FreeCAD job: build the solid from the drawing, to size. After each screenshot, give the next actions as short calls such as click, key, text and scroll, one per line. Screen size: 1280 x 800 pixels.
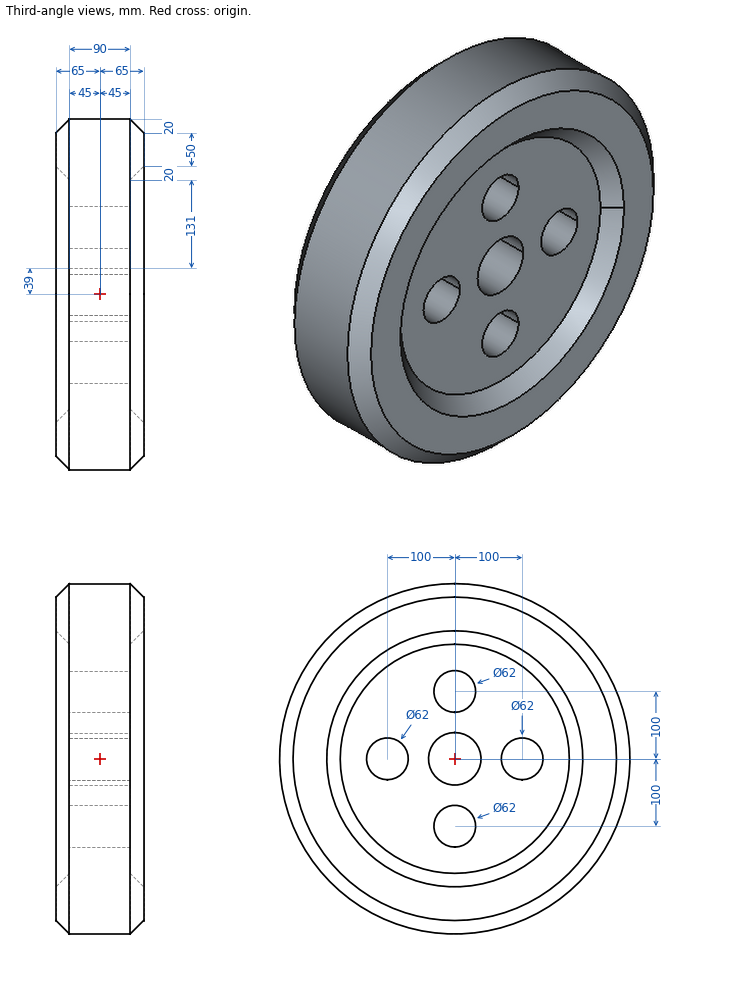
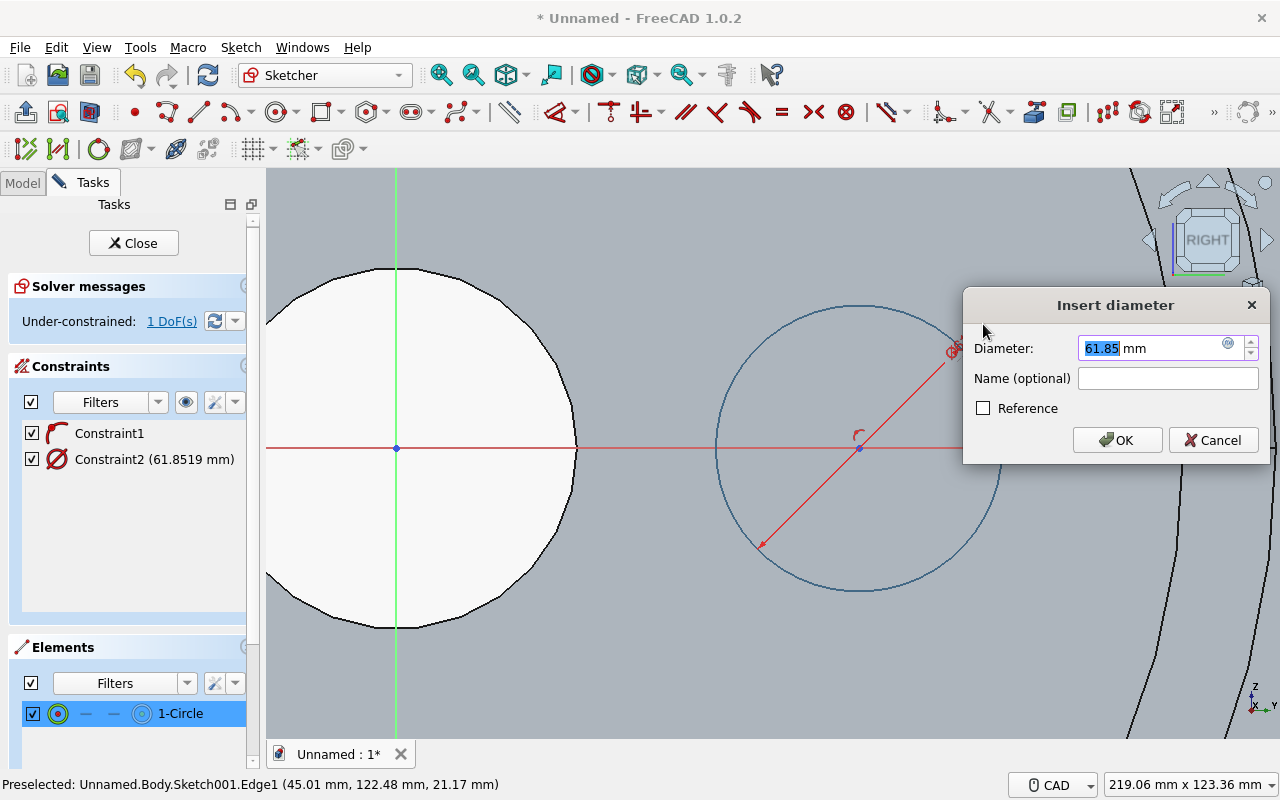
text(62)
key(Return)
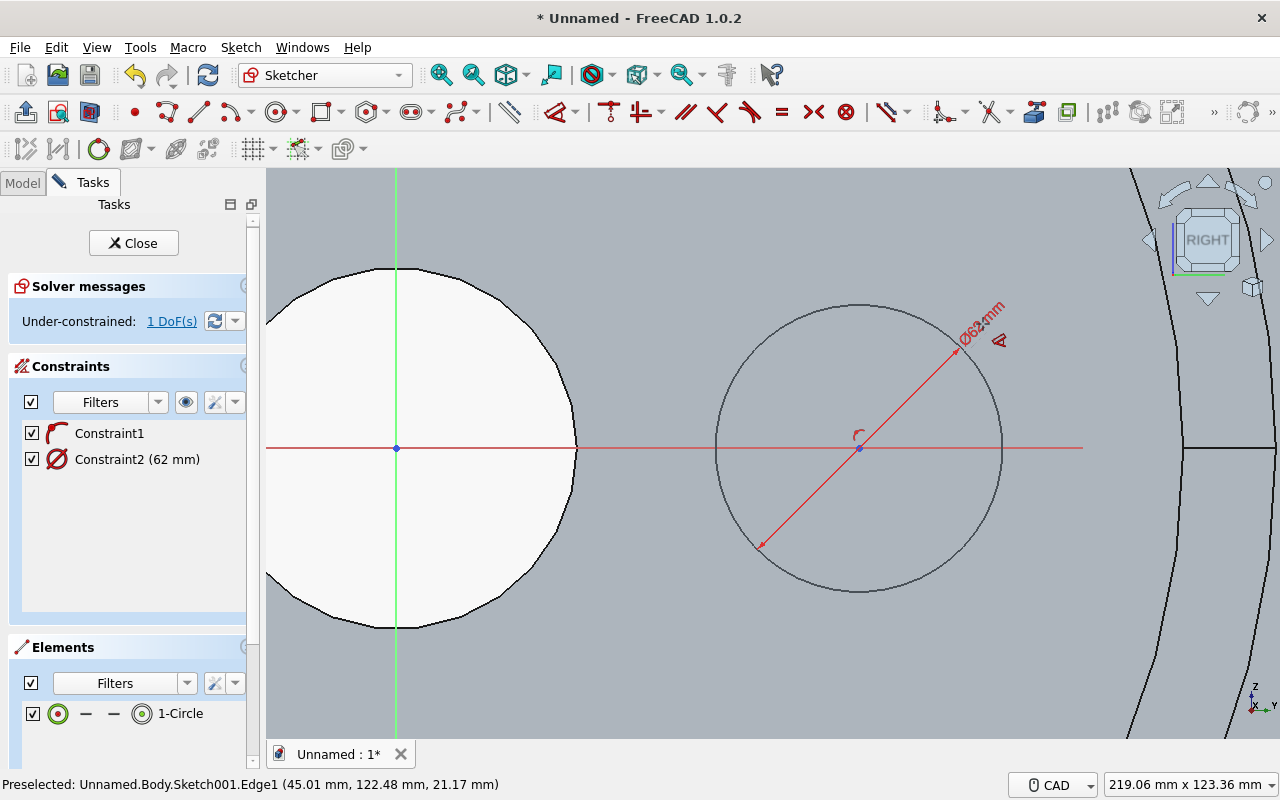
click(859, 448)
click(628, 482)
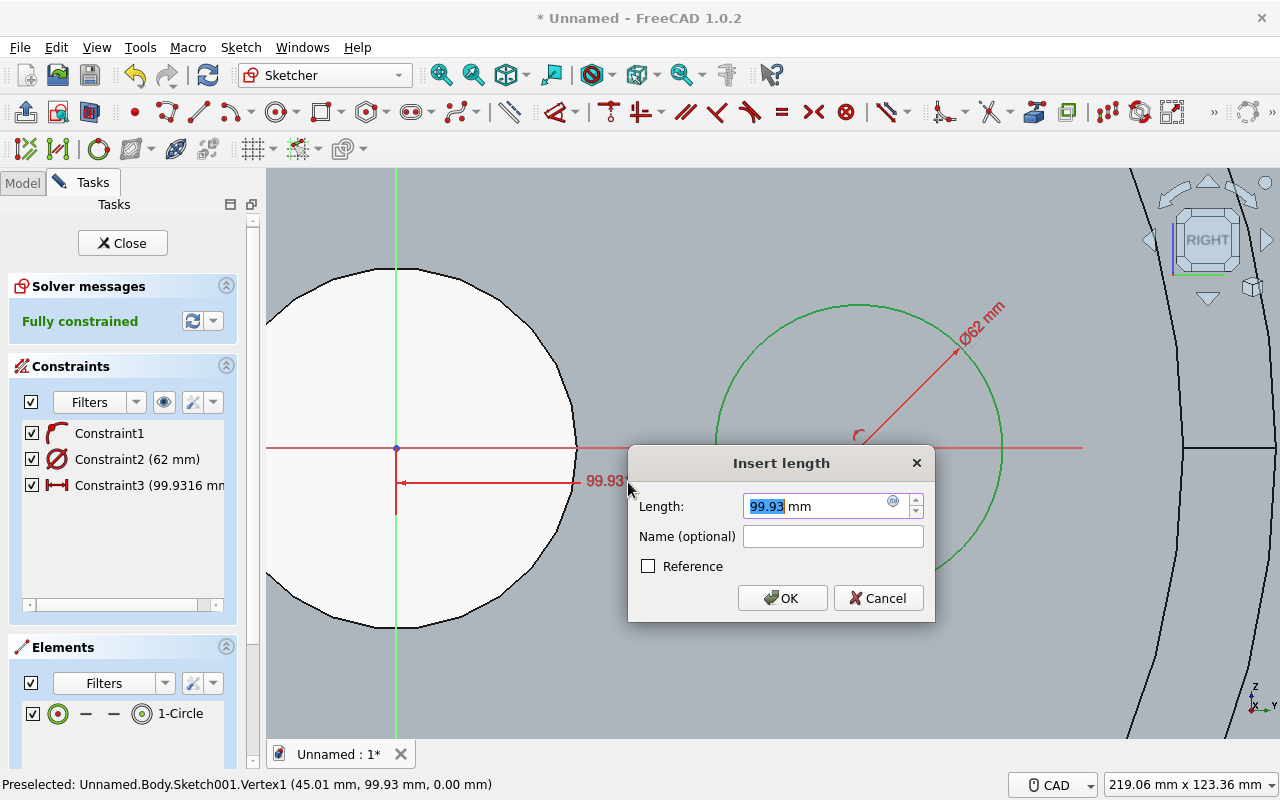
text(100)
key(Return)
key(Escape)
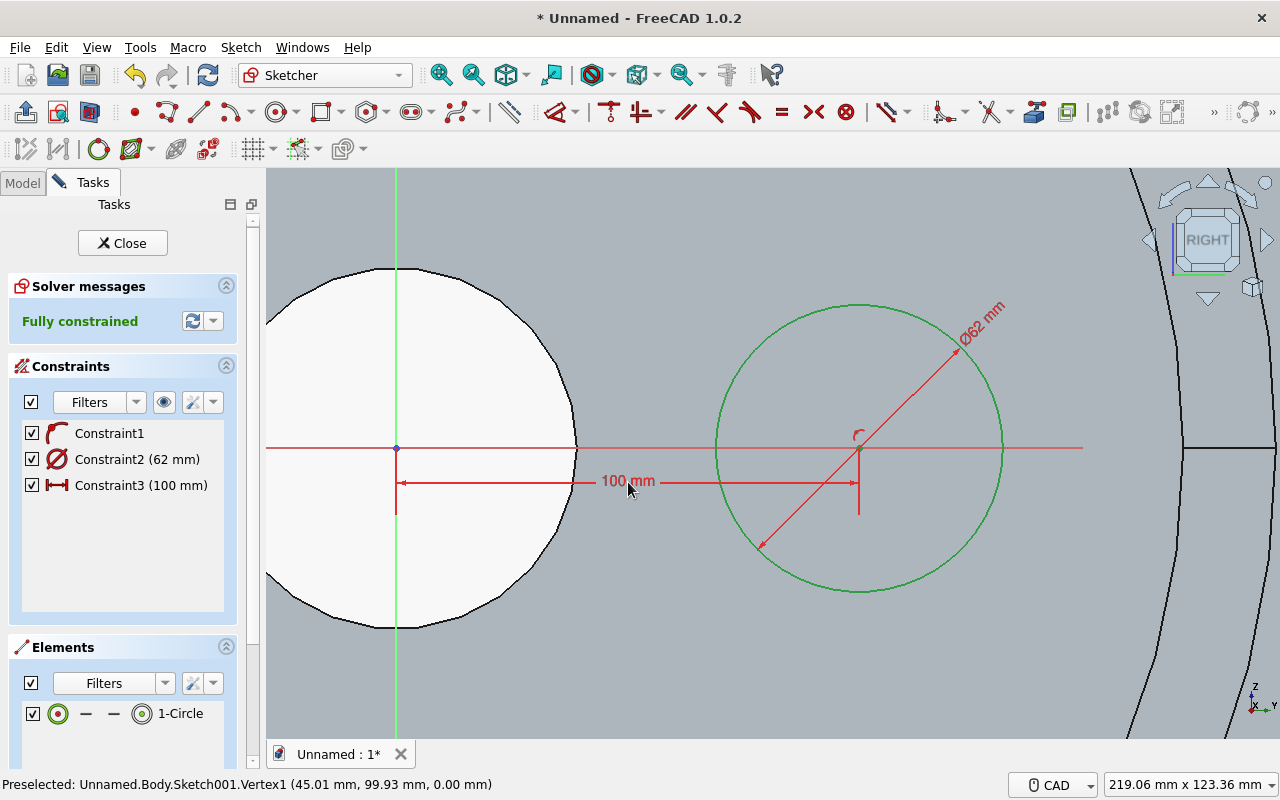
click(123, 243)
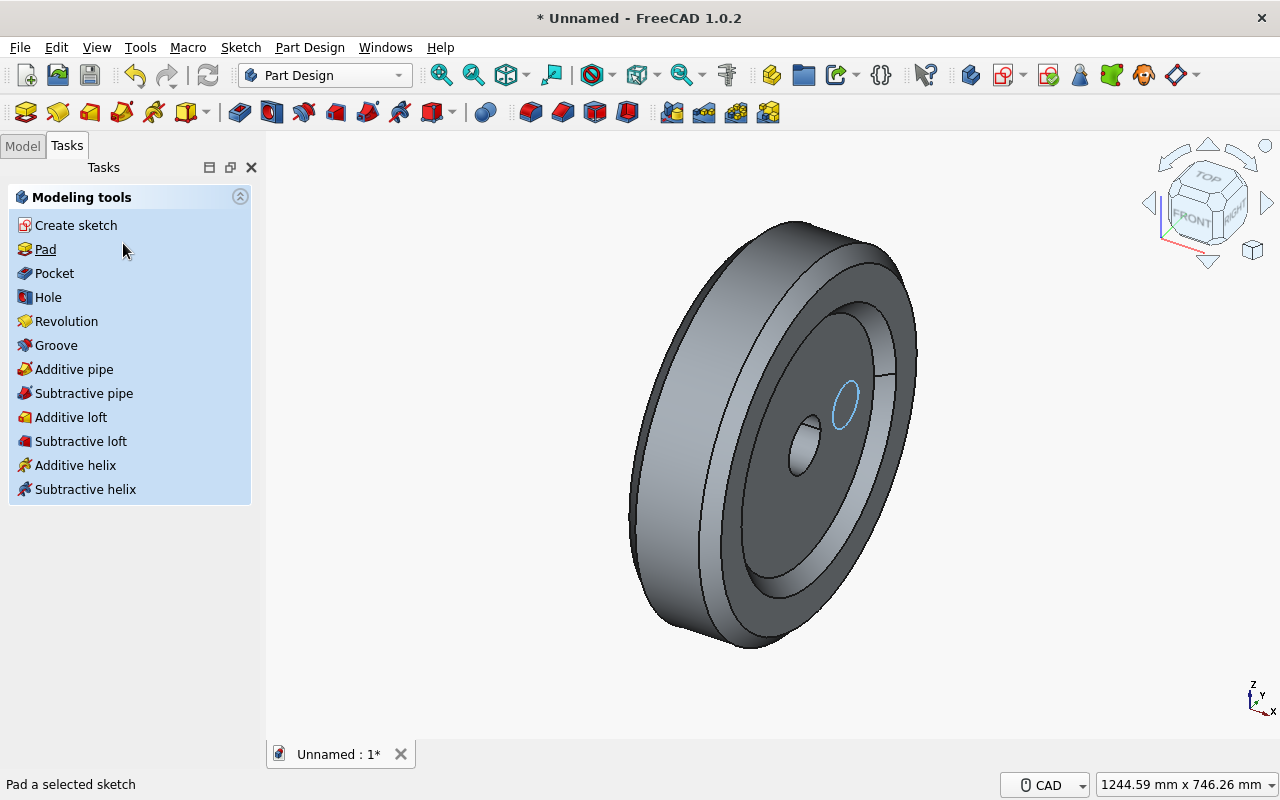
click(240, 112)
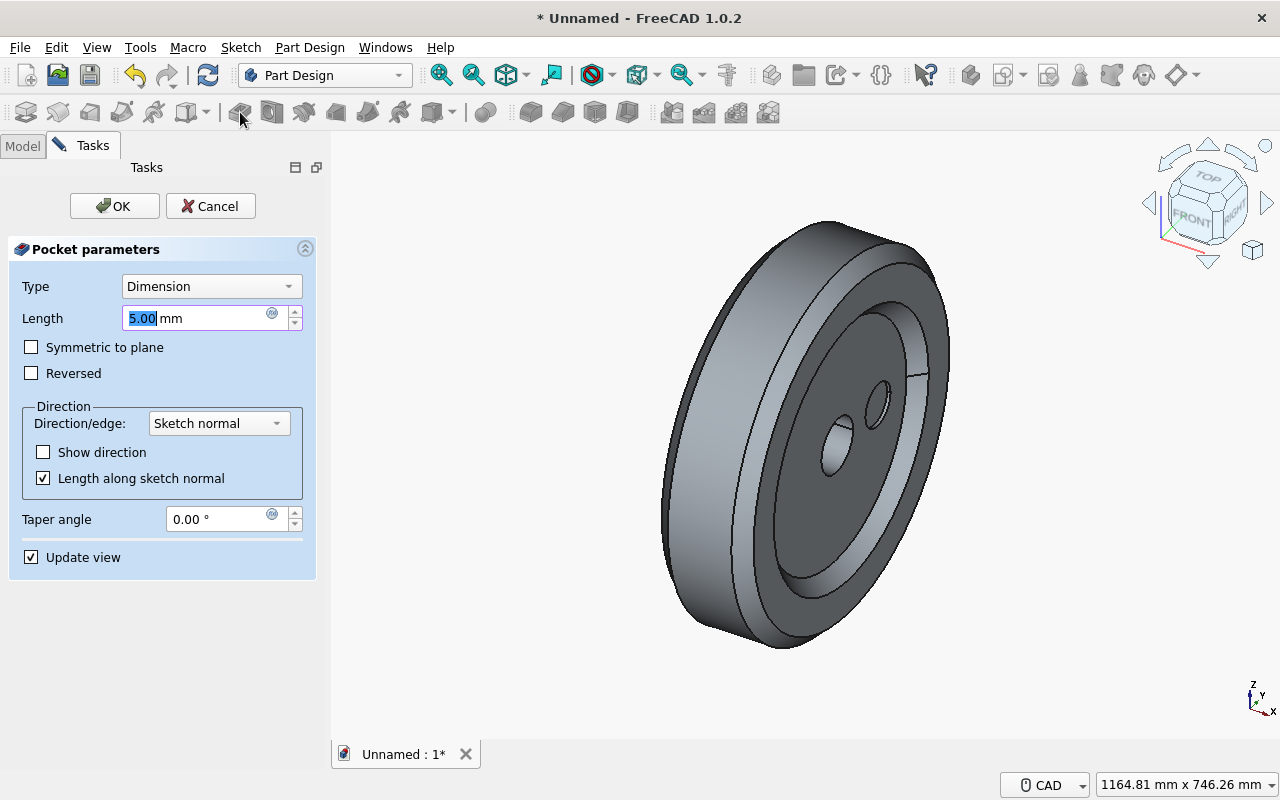
click(212, 286)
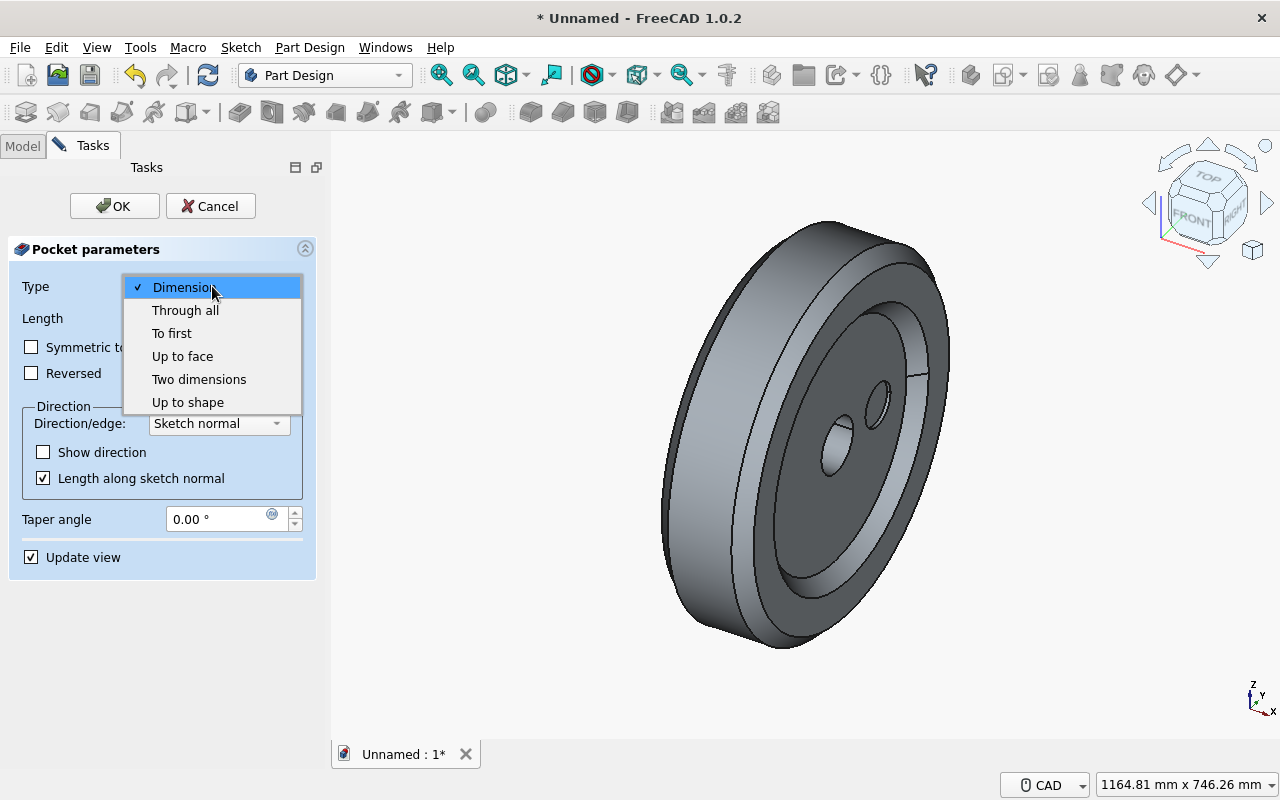
click(212, 334)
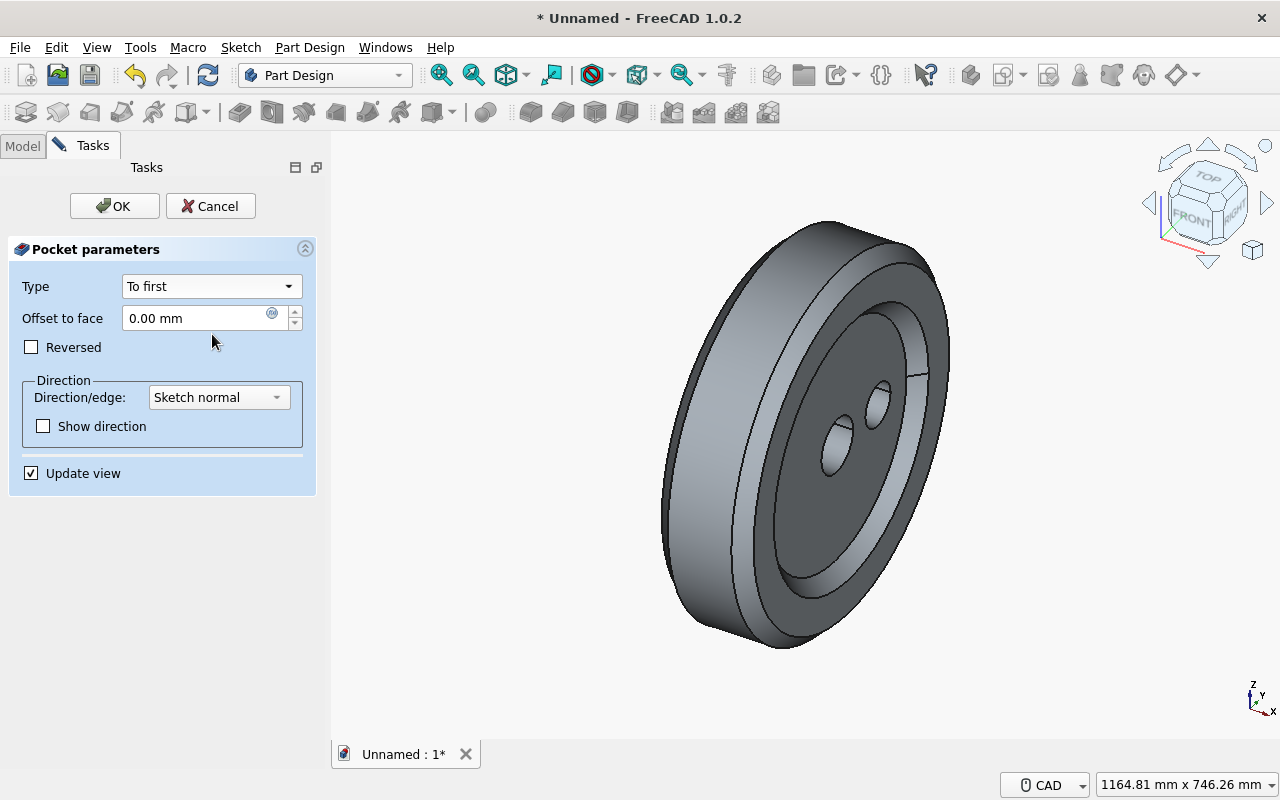
click(115, 206)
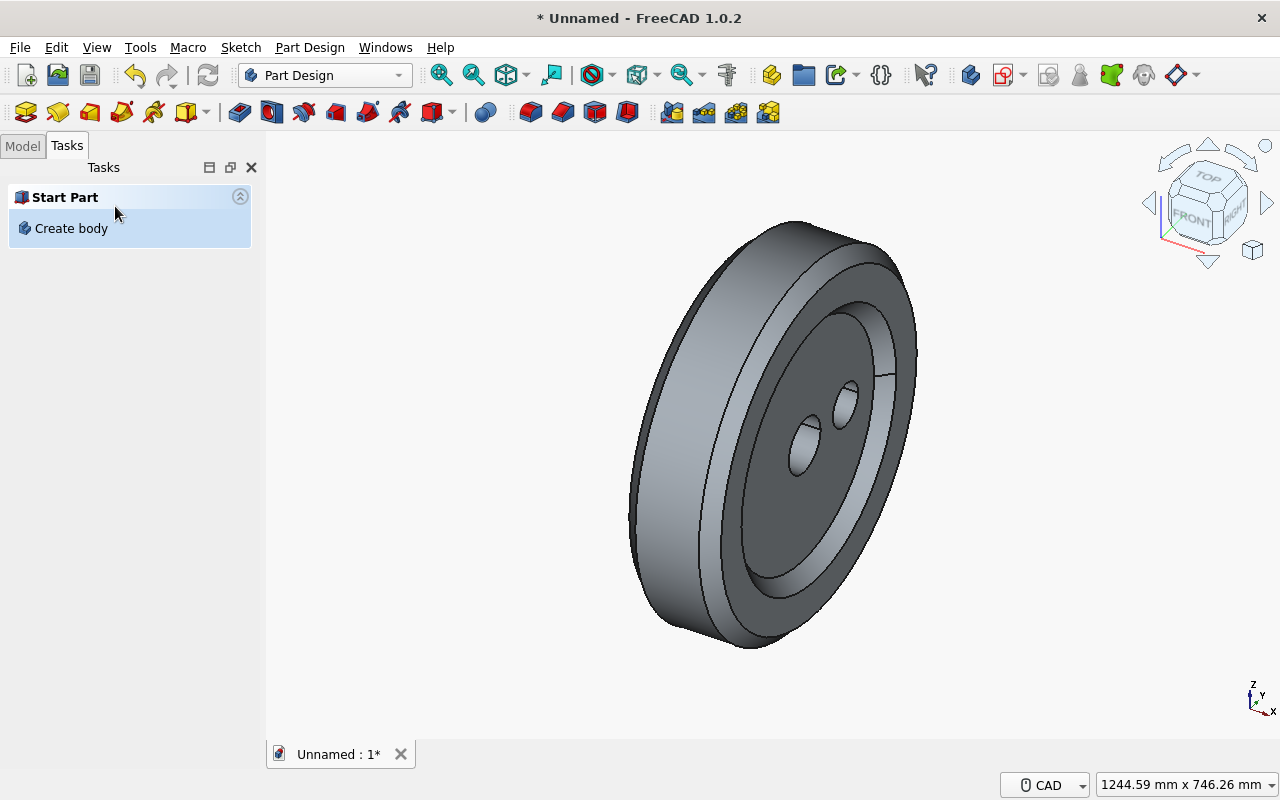
click(825, 490)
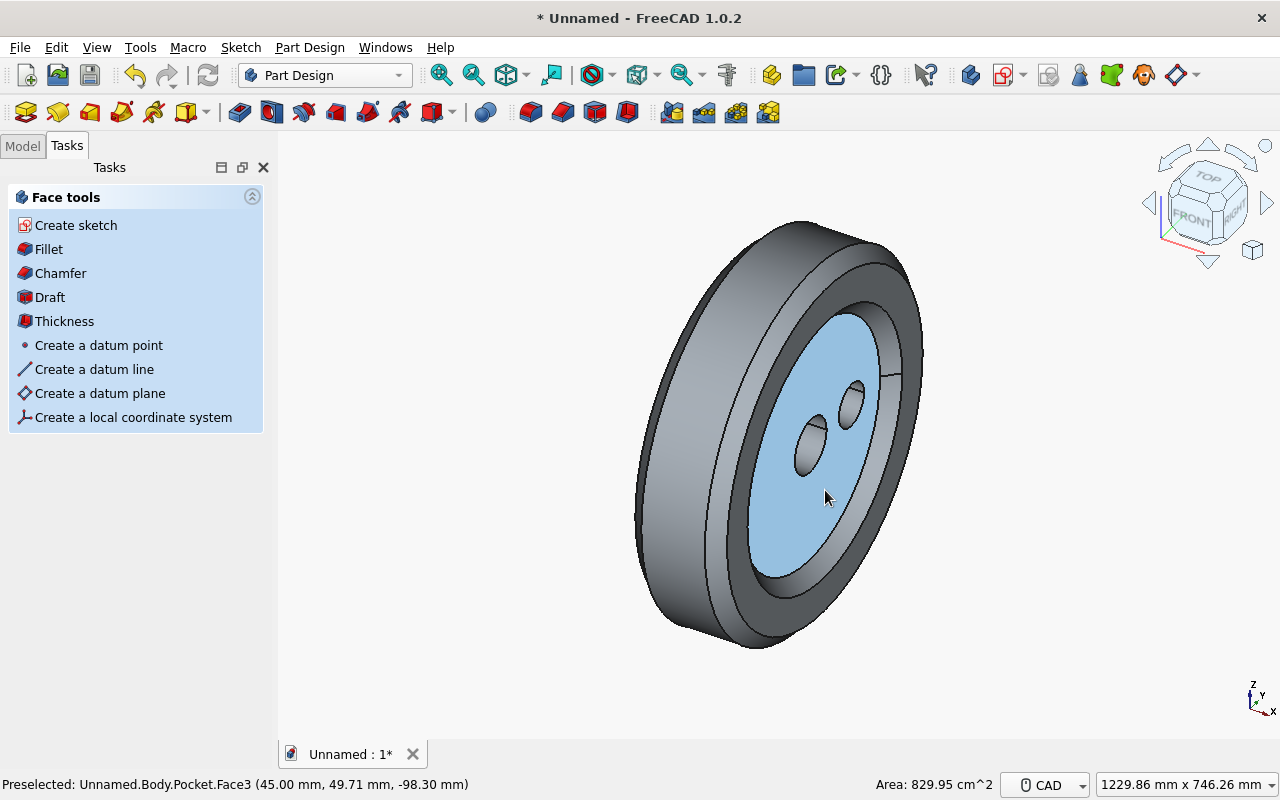
click(1004, 76)